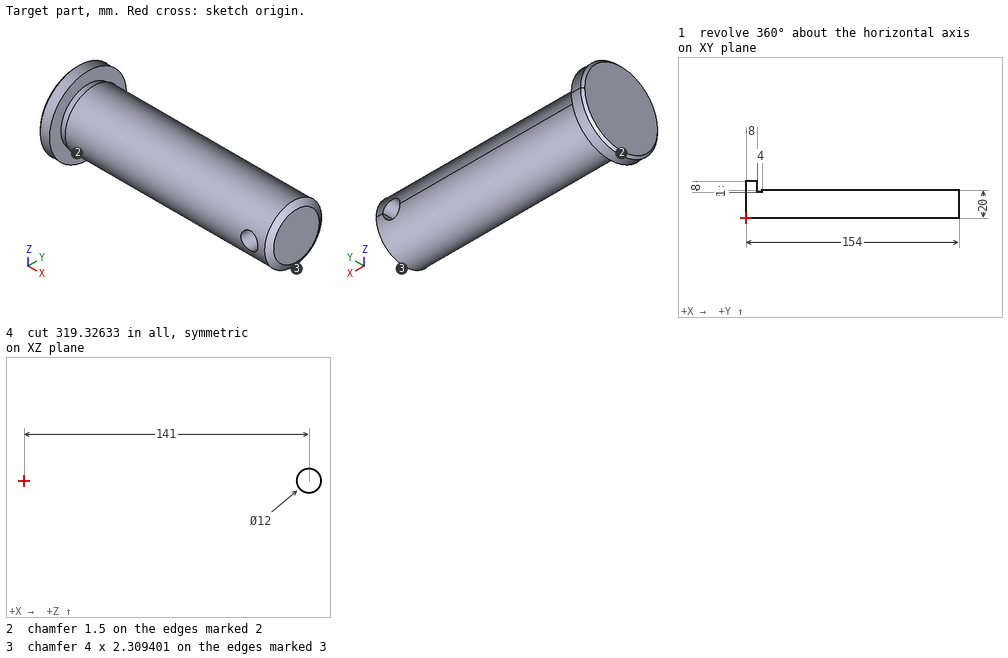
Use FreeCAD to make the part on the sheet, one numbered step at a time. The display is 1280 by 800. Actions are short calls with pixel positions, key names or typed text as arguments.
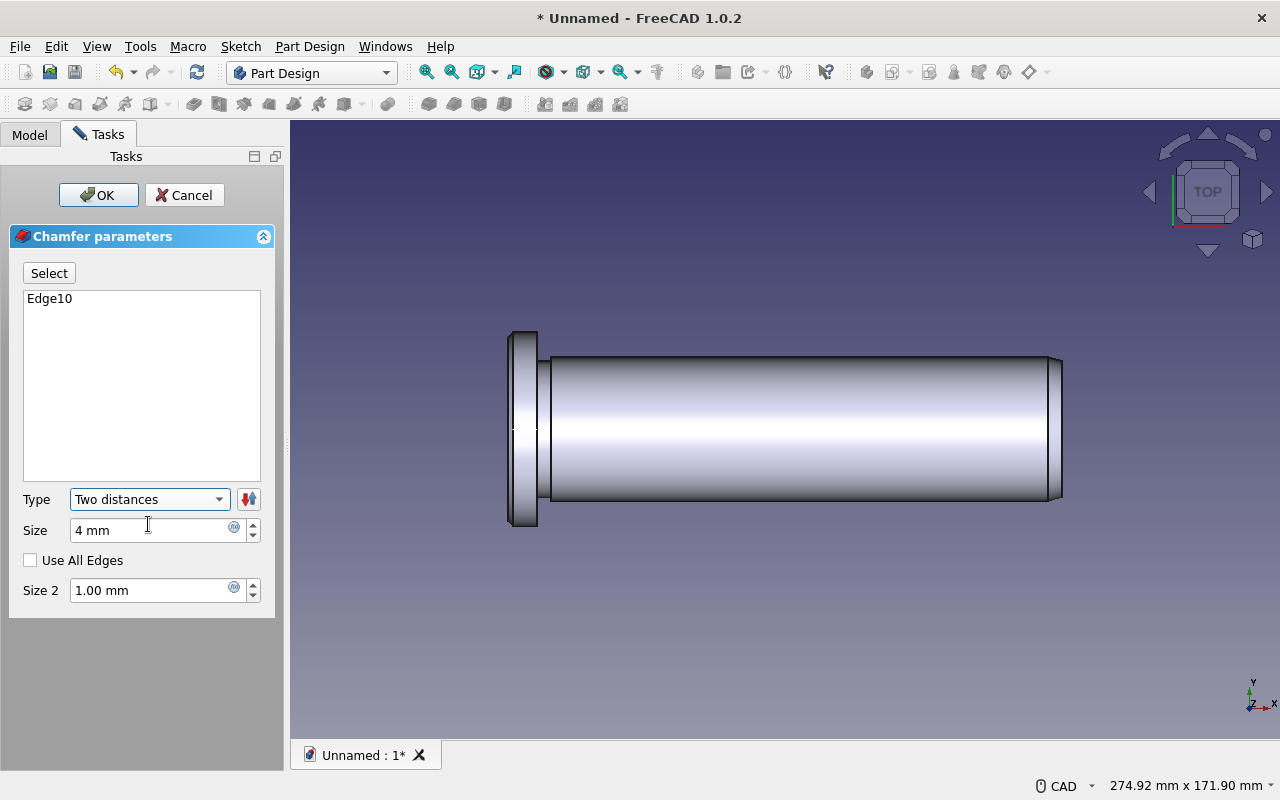
triple_click(158, 590)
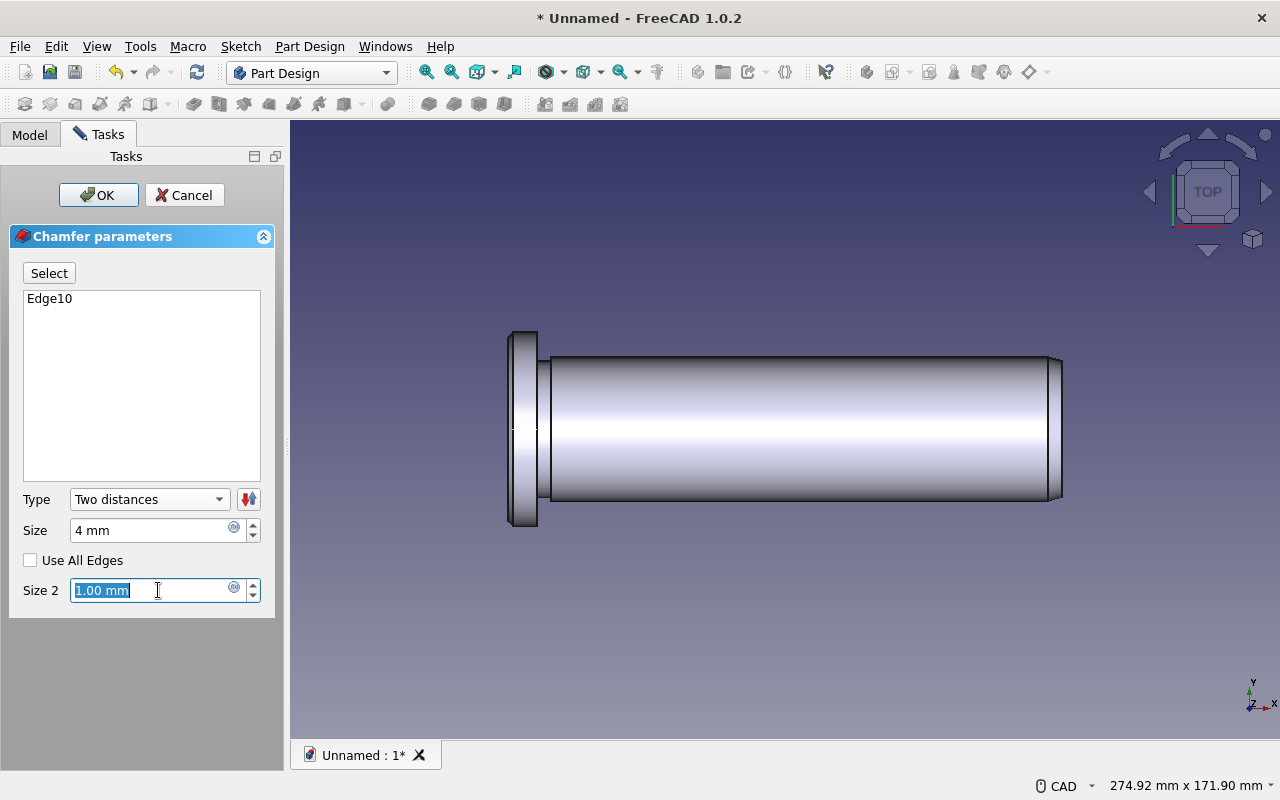
text(2.309401)
key(Tab)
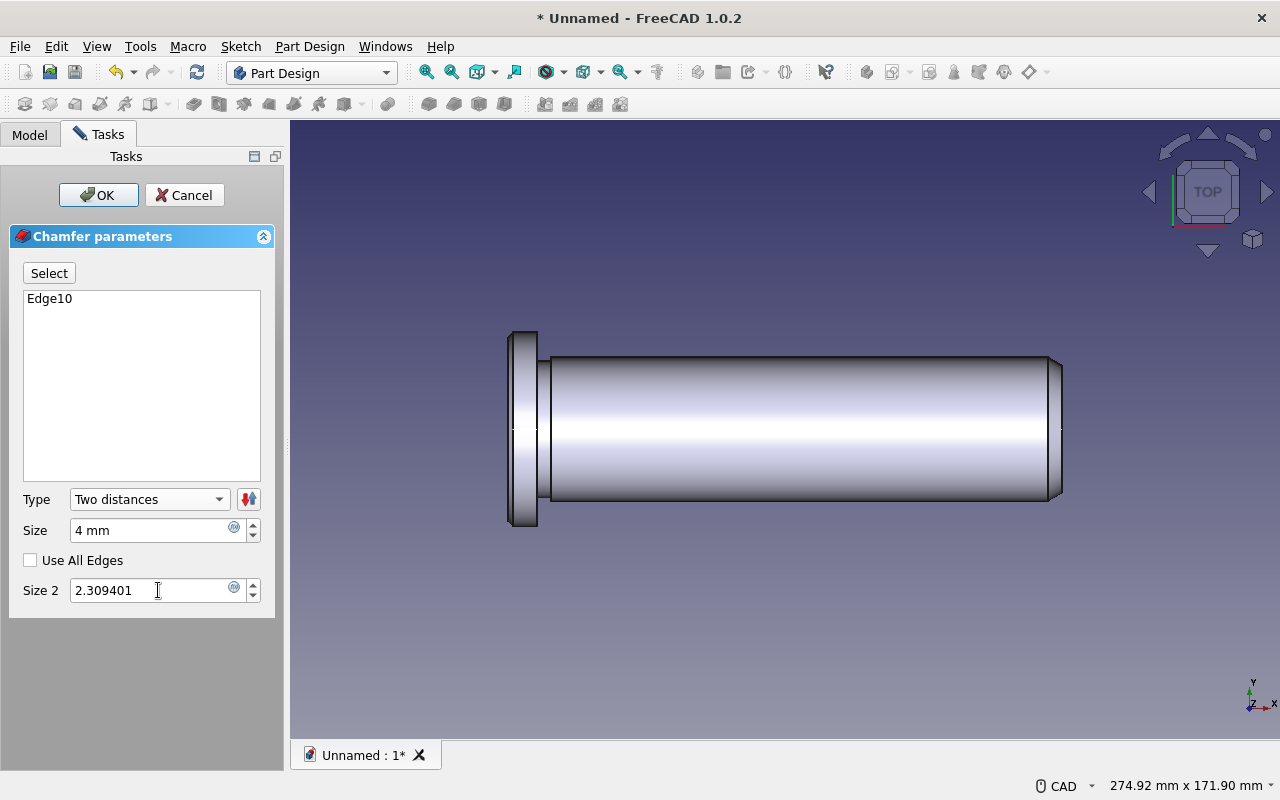
click(249, 500)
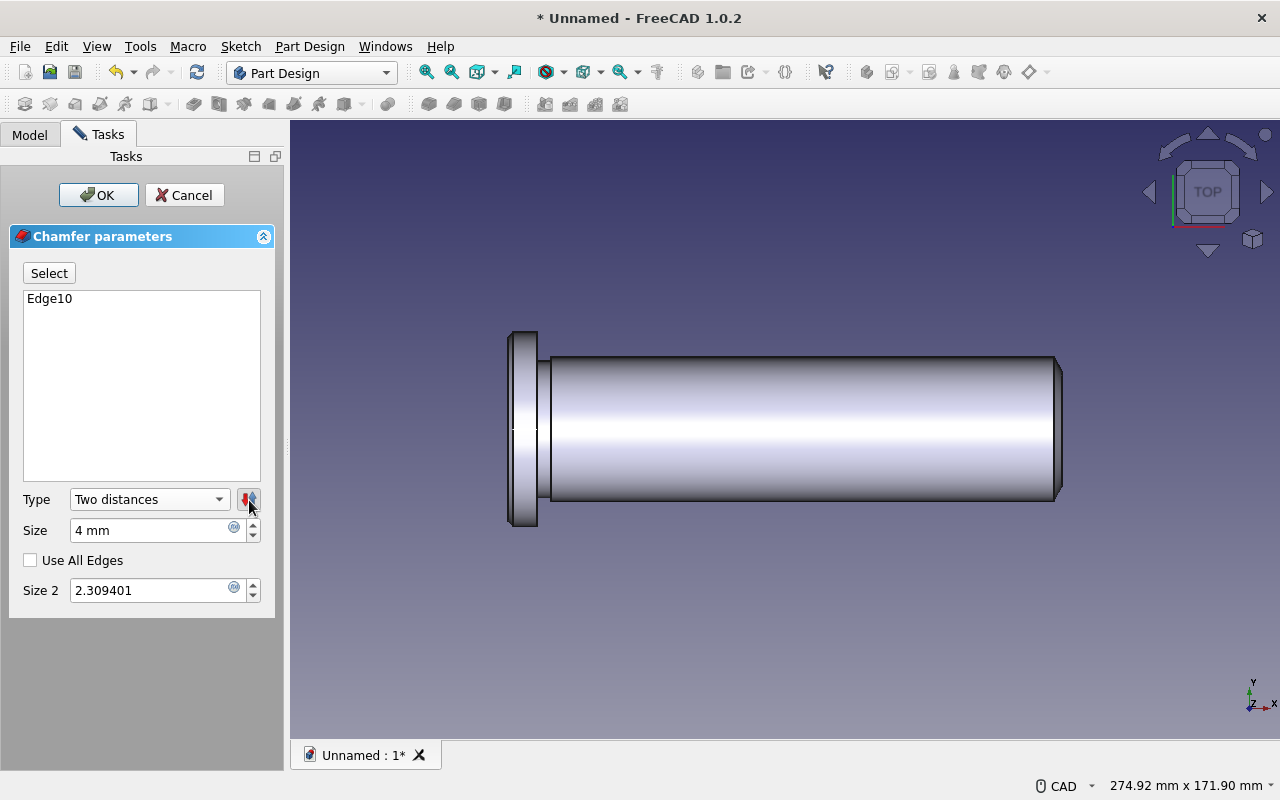
click(99, 195)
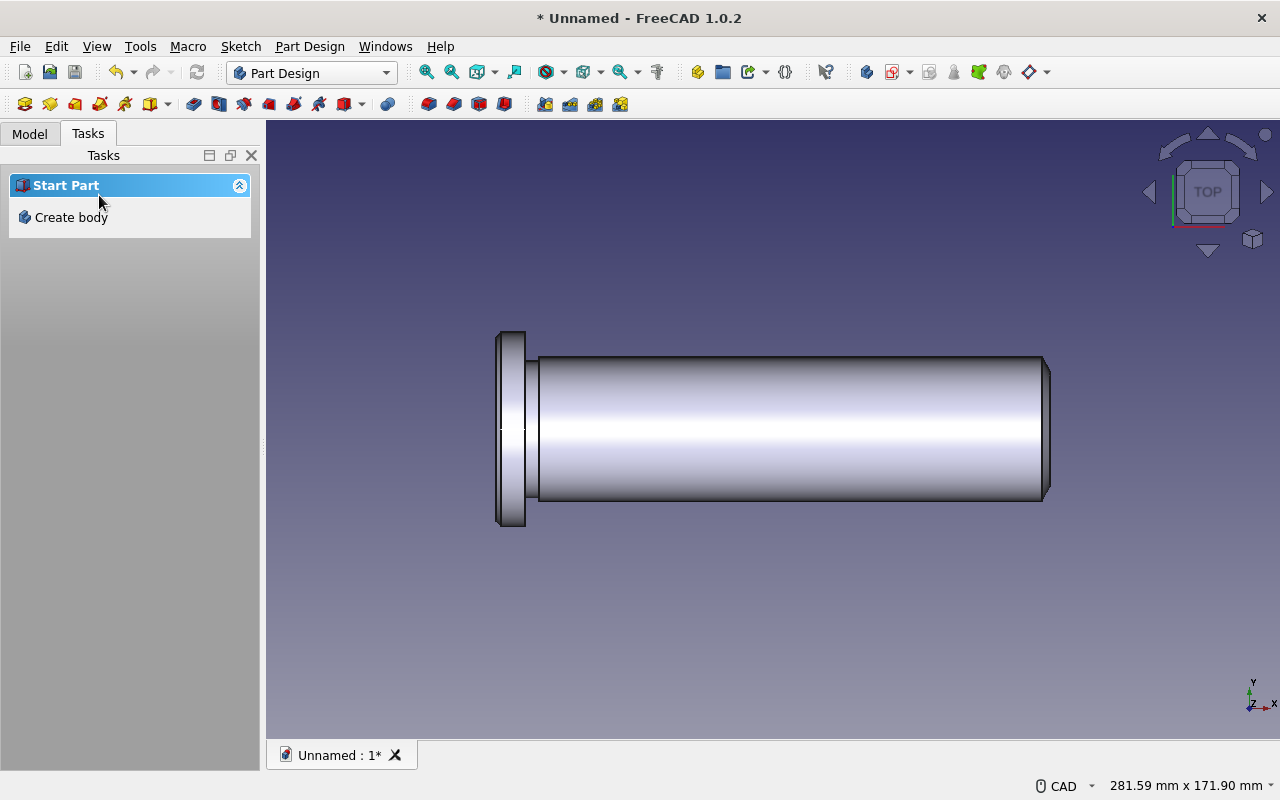
click(892, 72)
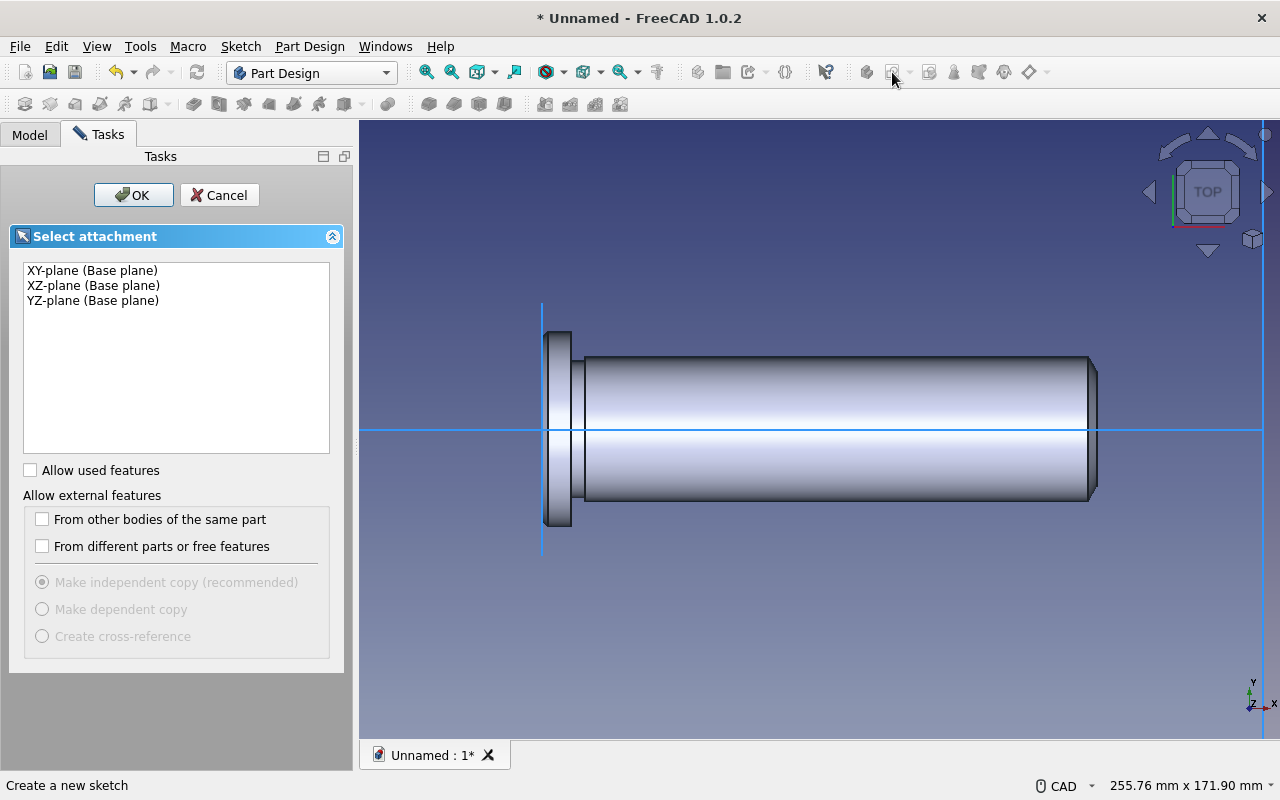
click(84, 286)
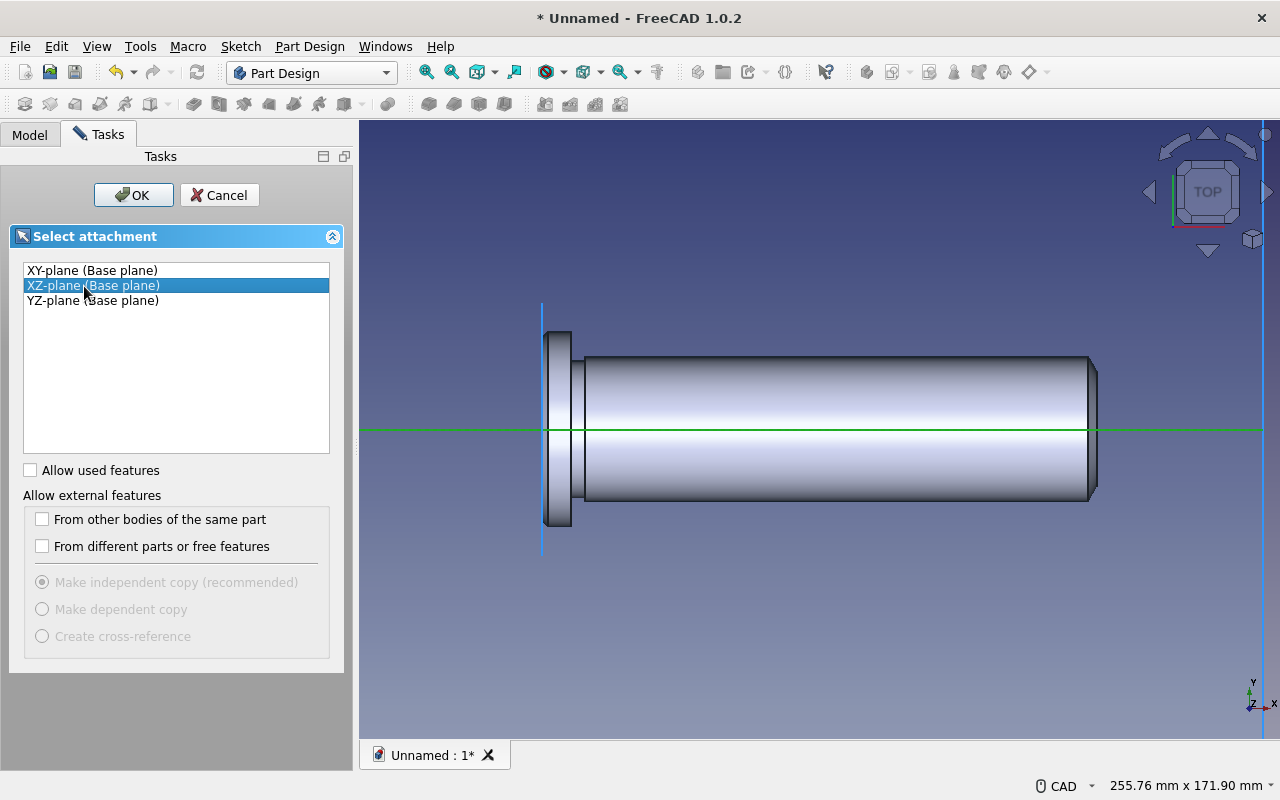
click(134, 195)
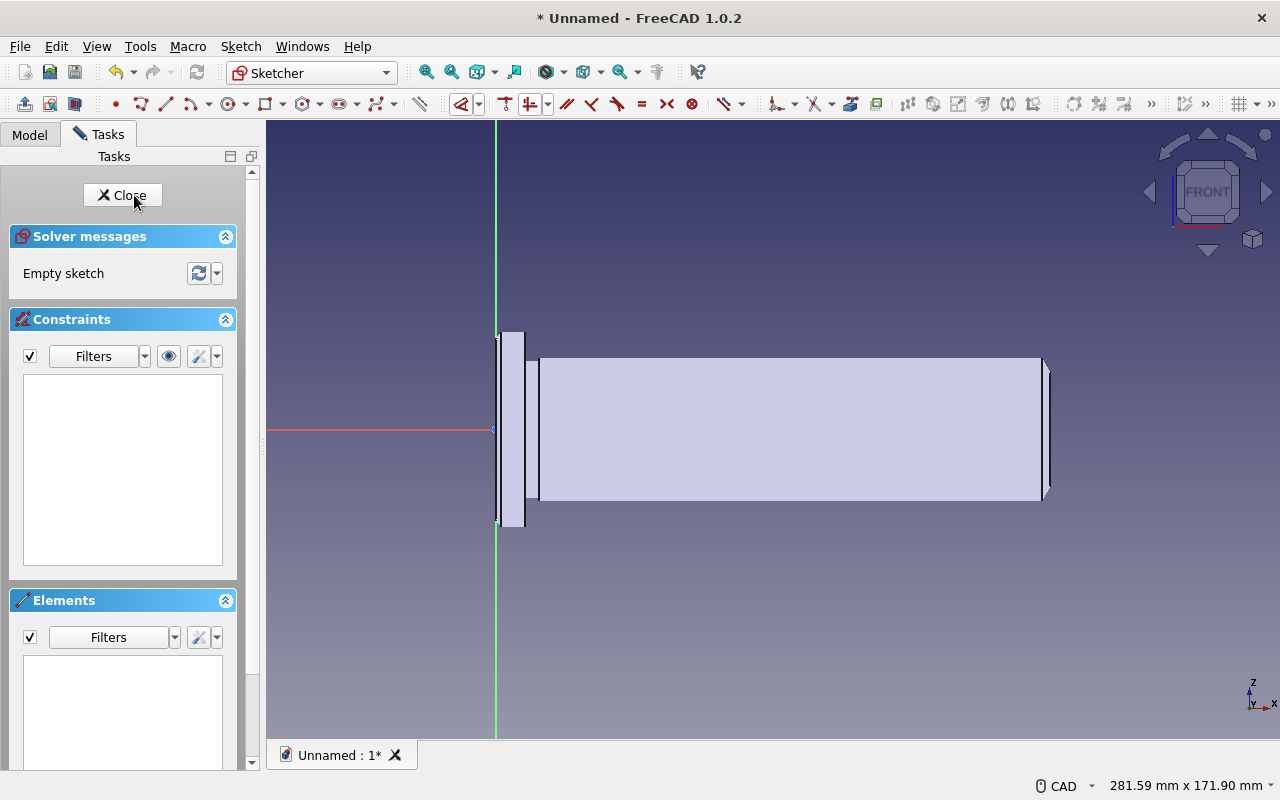
click(75, 104)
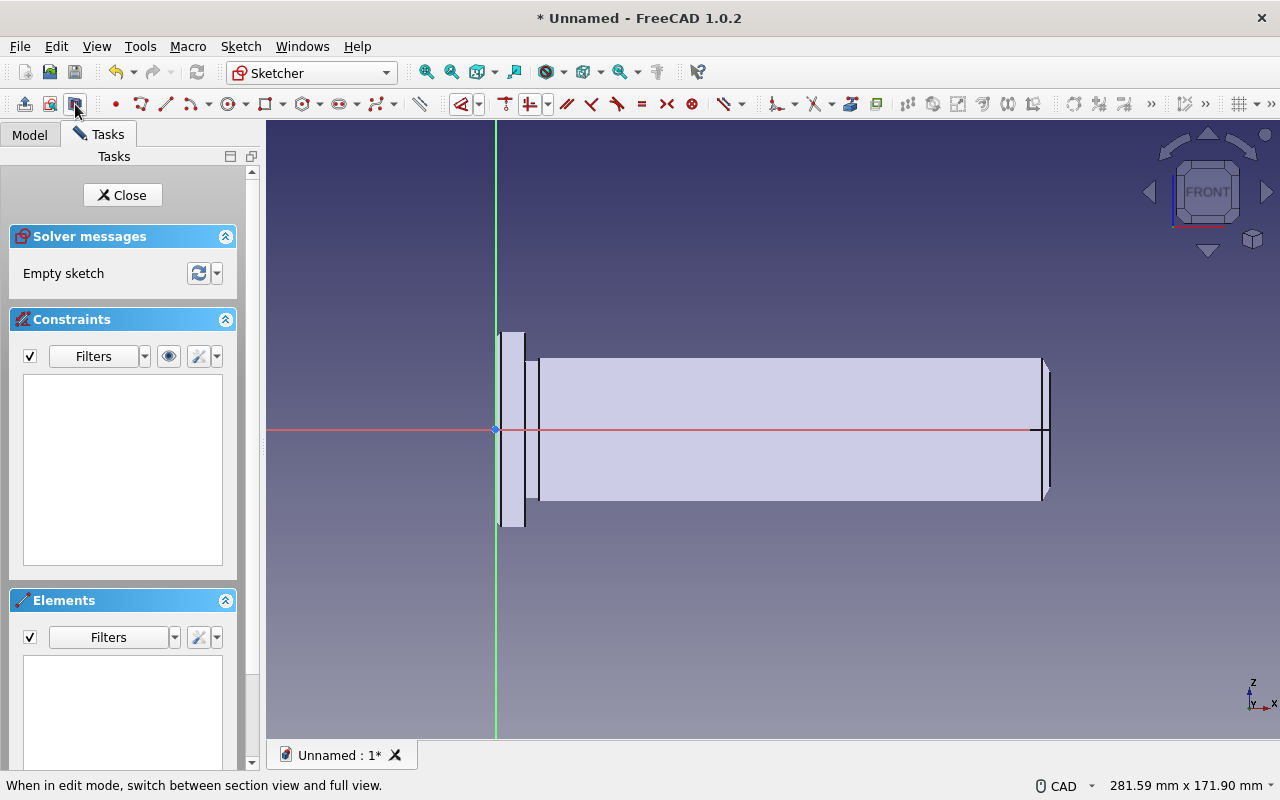
scroll(1041, 429, up, 11)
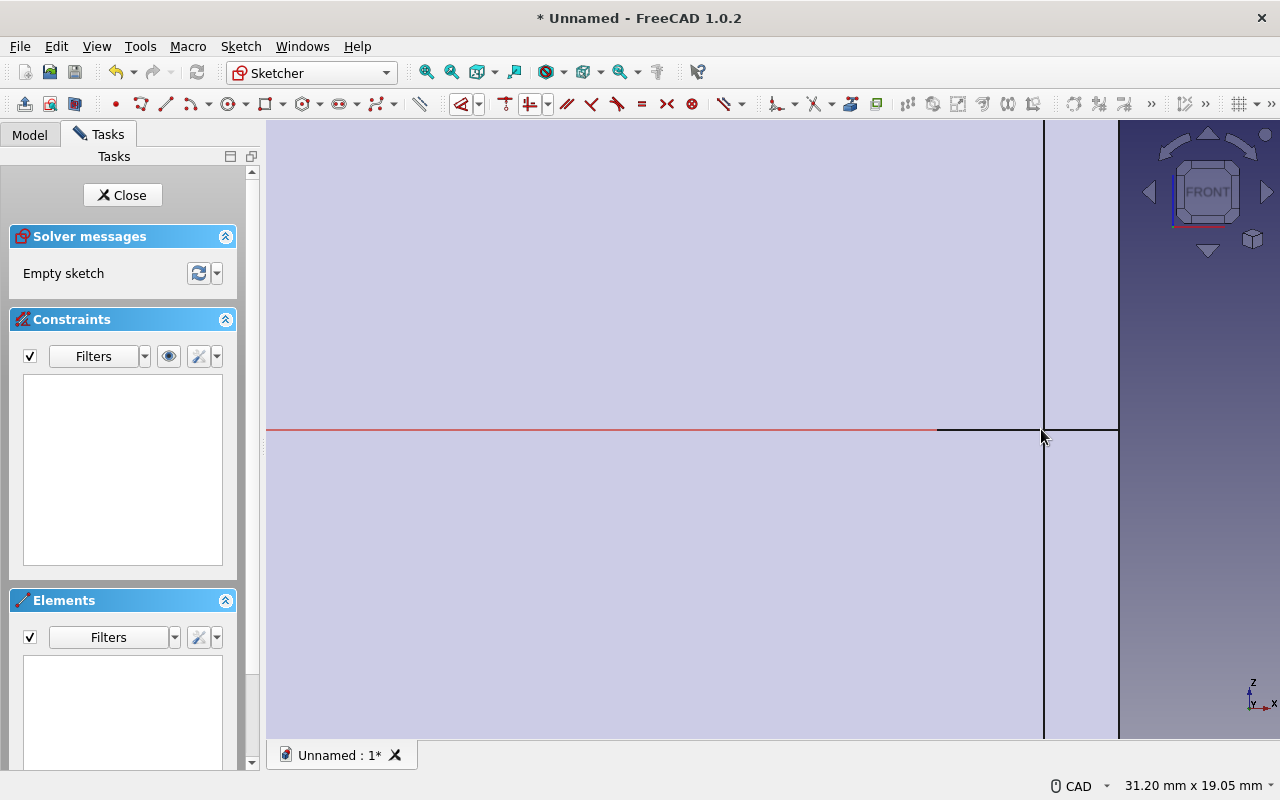
click(228, 104)